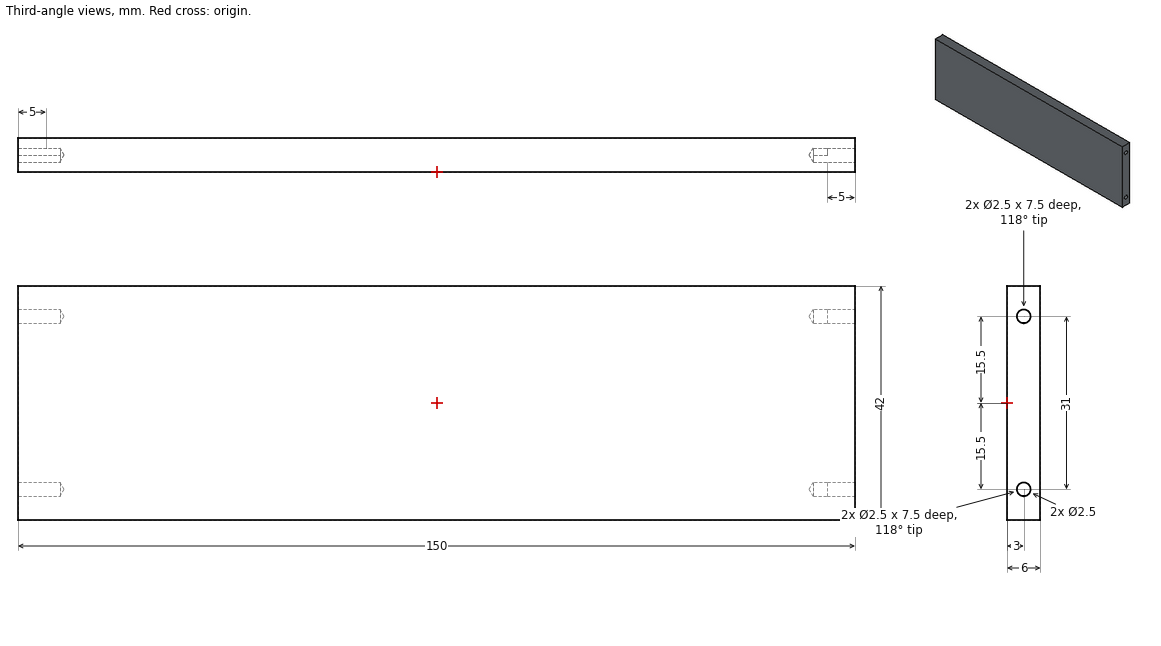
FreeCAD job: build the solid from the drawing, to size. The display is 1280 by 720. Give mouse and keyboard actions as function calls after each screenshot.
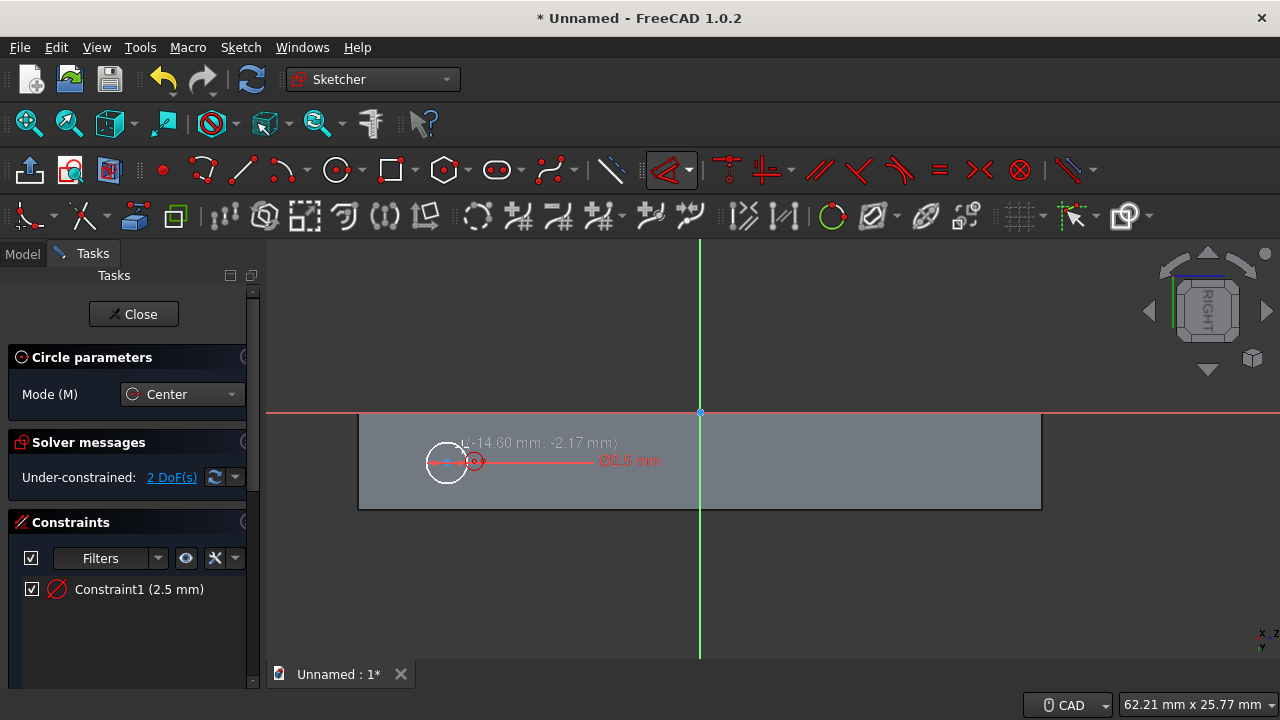
click(953, 462)
move(967, 447)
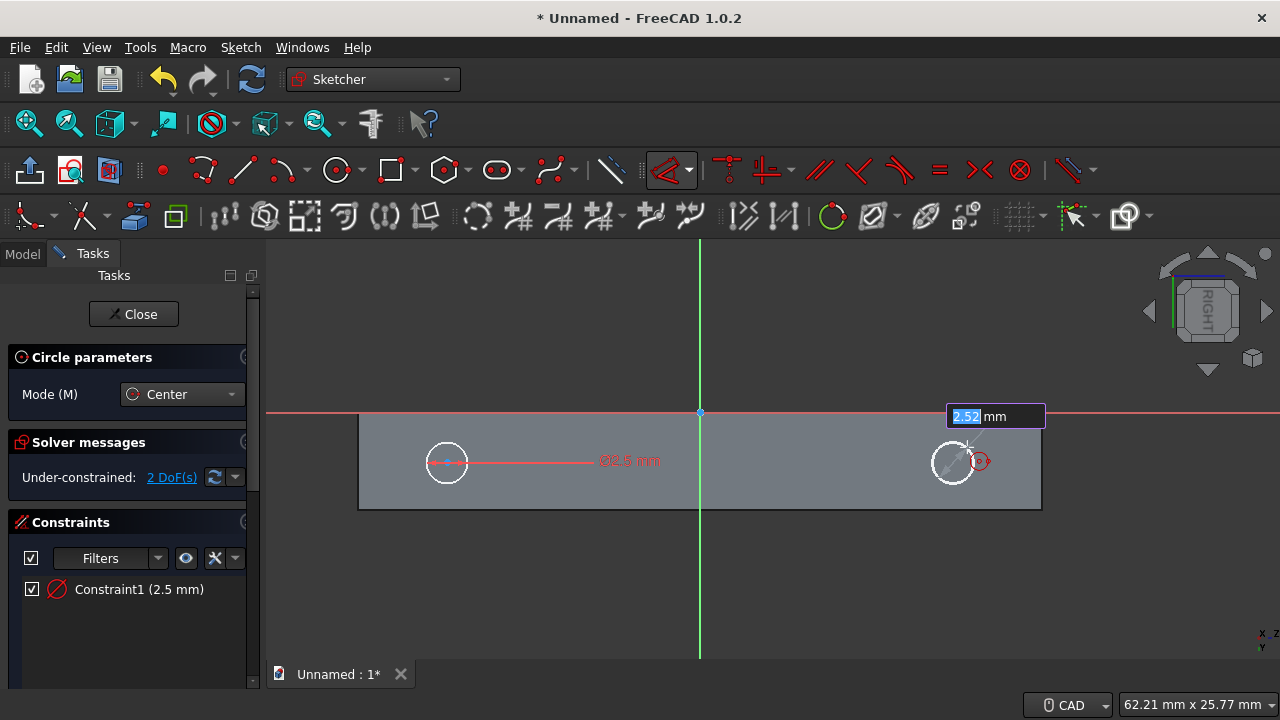
text(2.5)
key(Return)
key(Escape)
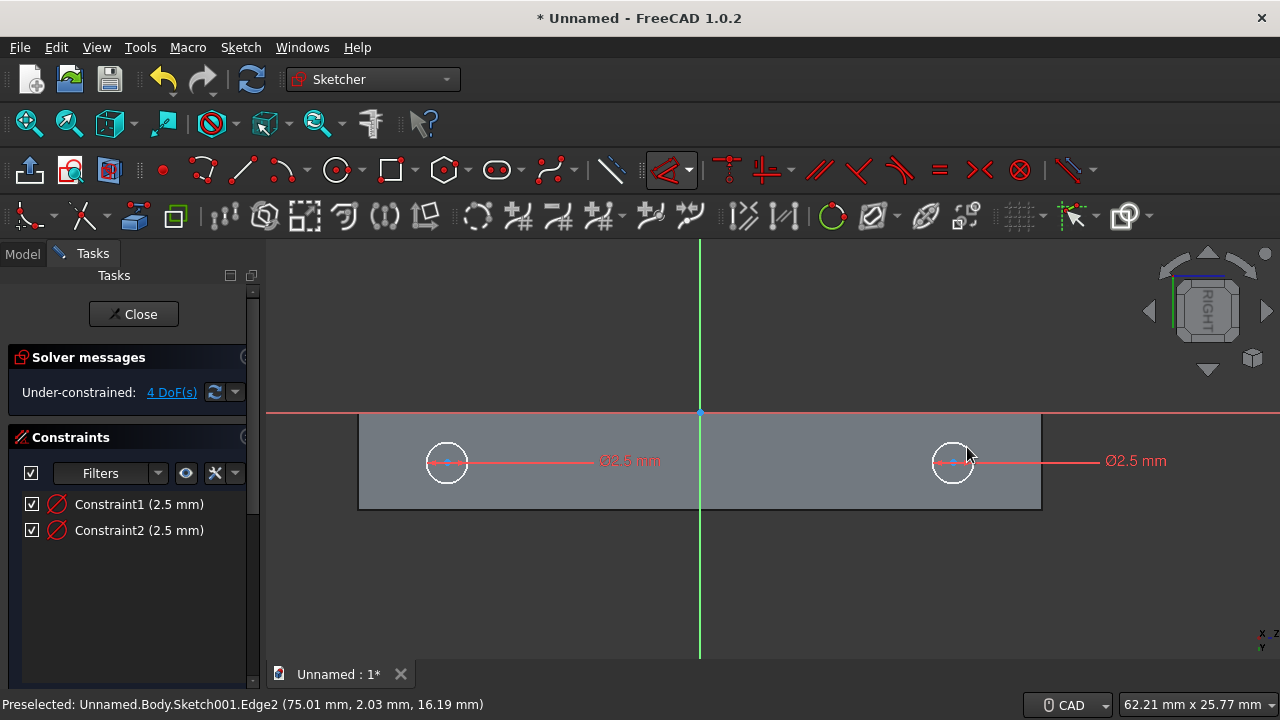
click(447, 463)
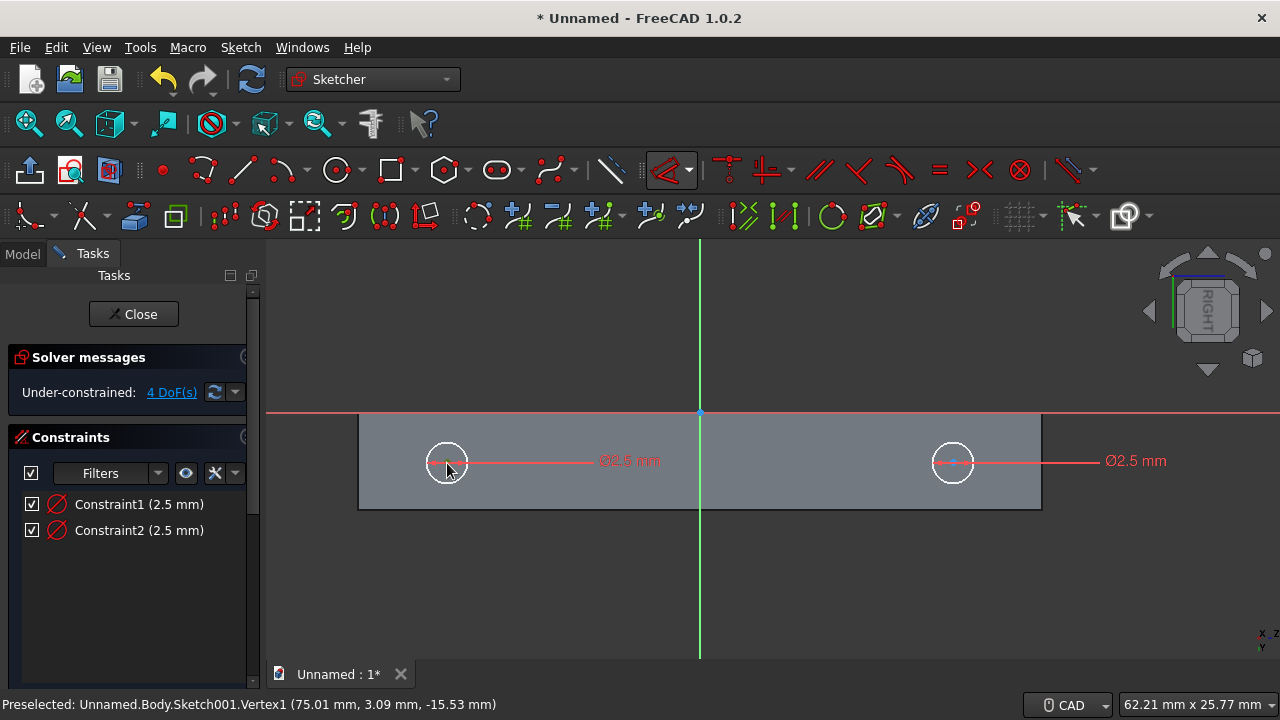
click(953, 463)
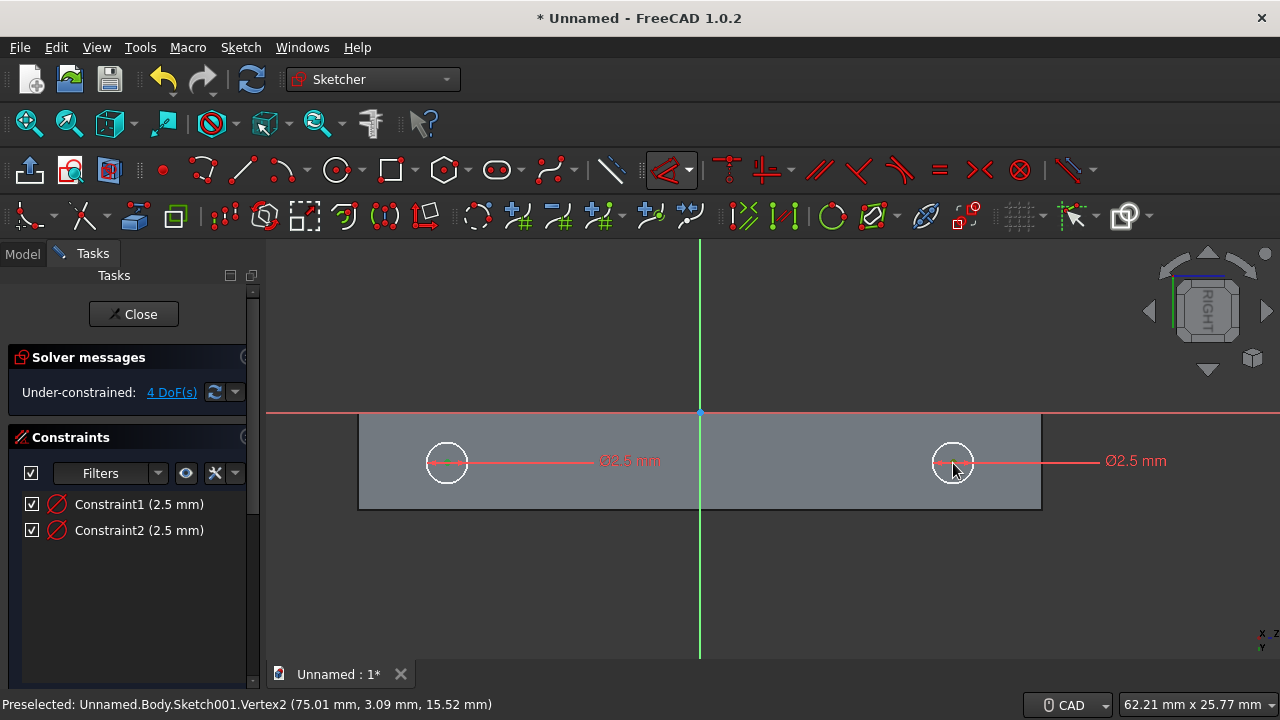
key(h)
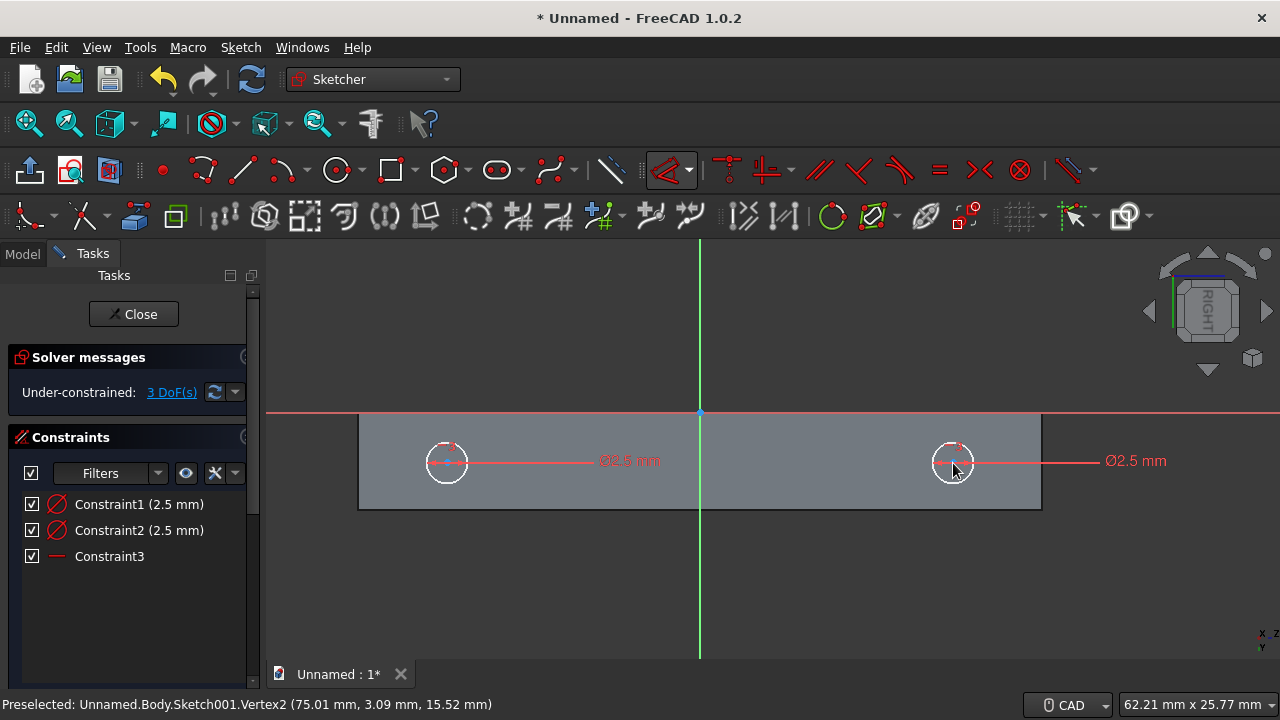
click(666, 170)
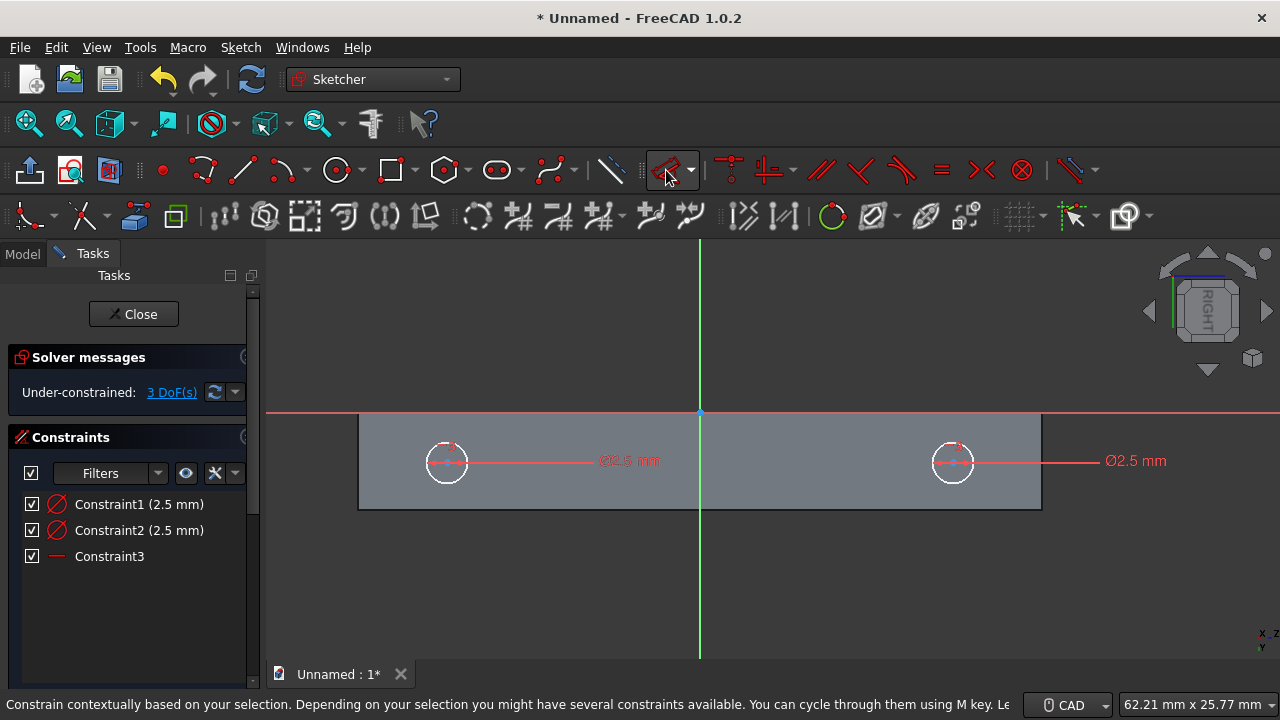
click(447, 463)
click(413, 438)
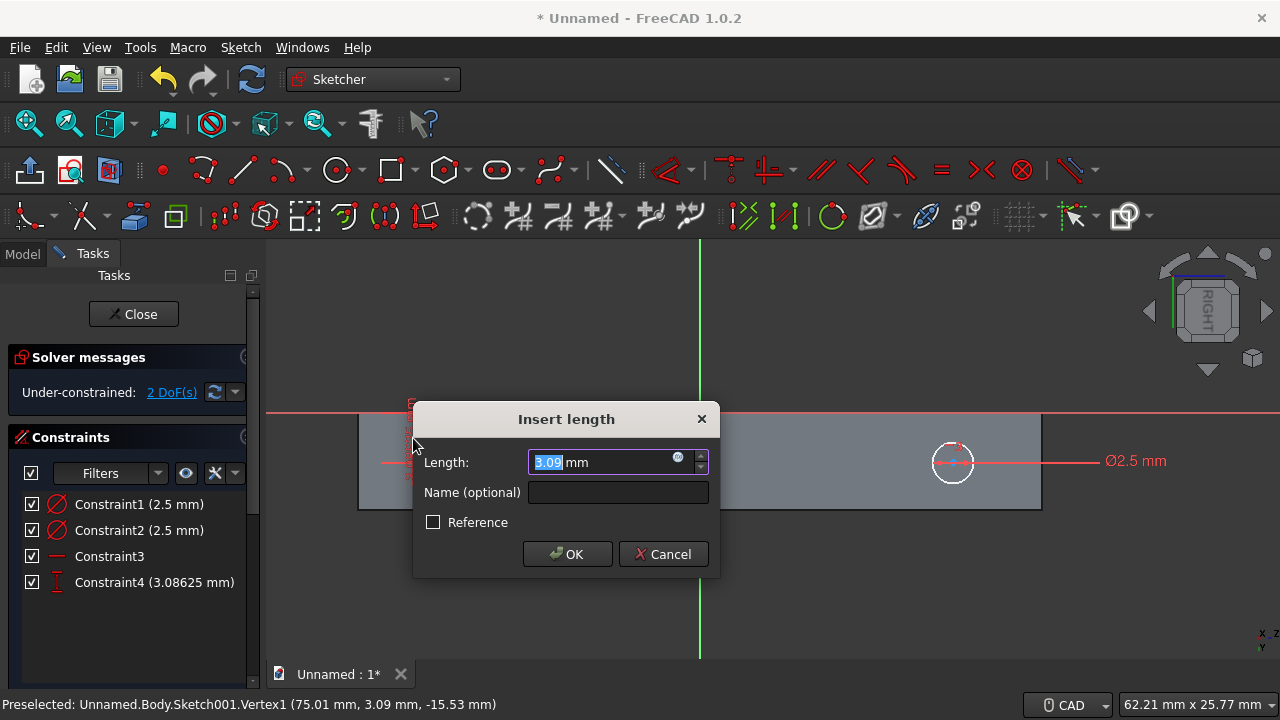
text(3)
key(Return)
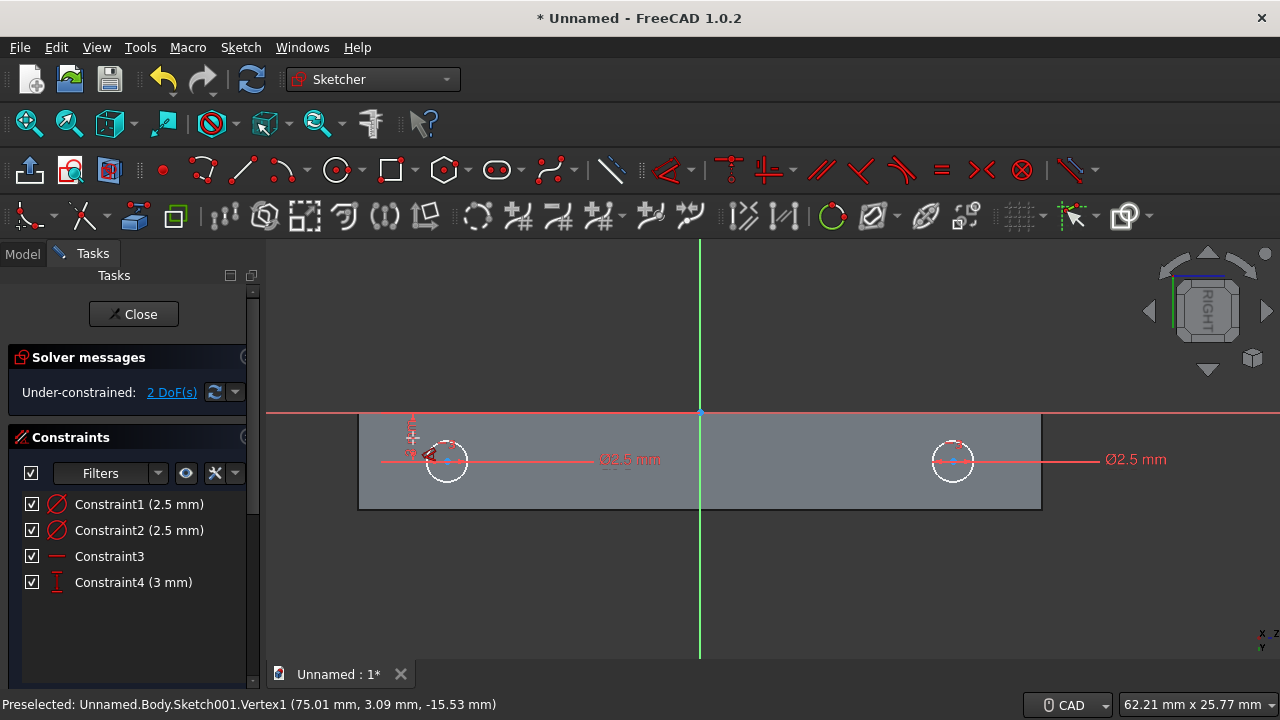
click(447, 462)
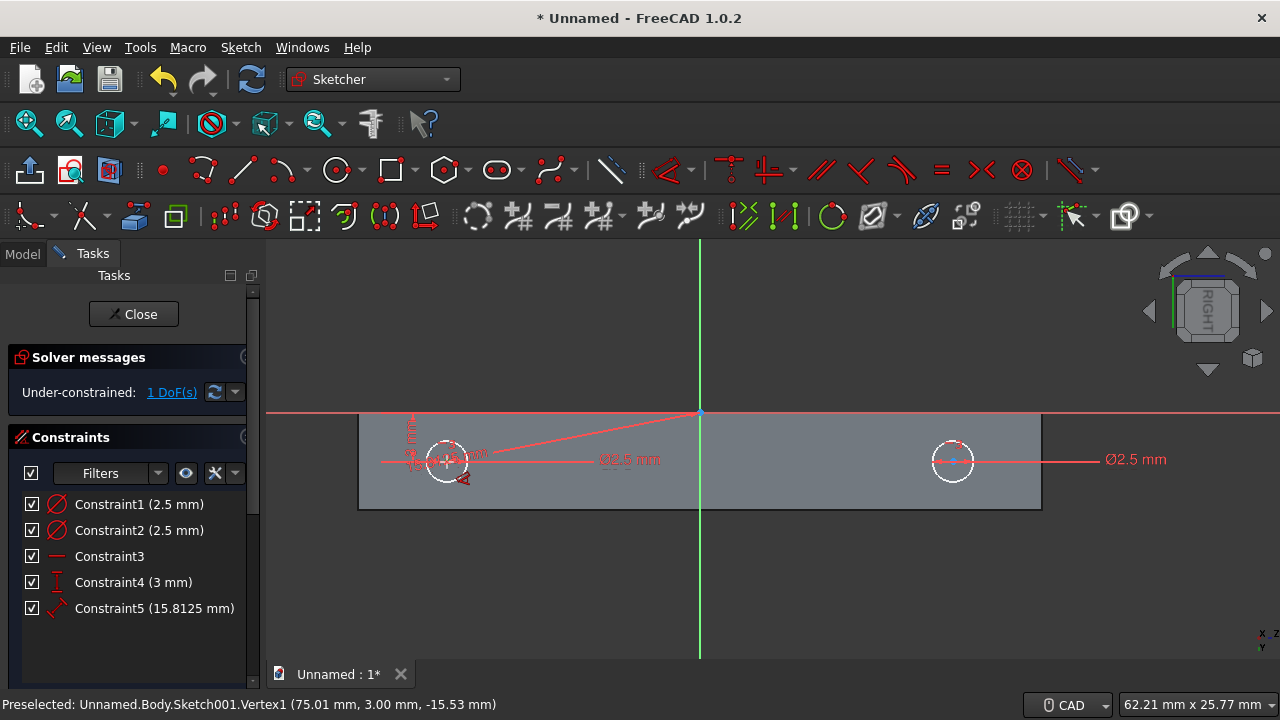
click(953, 462)
click(584, 496)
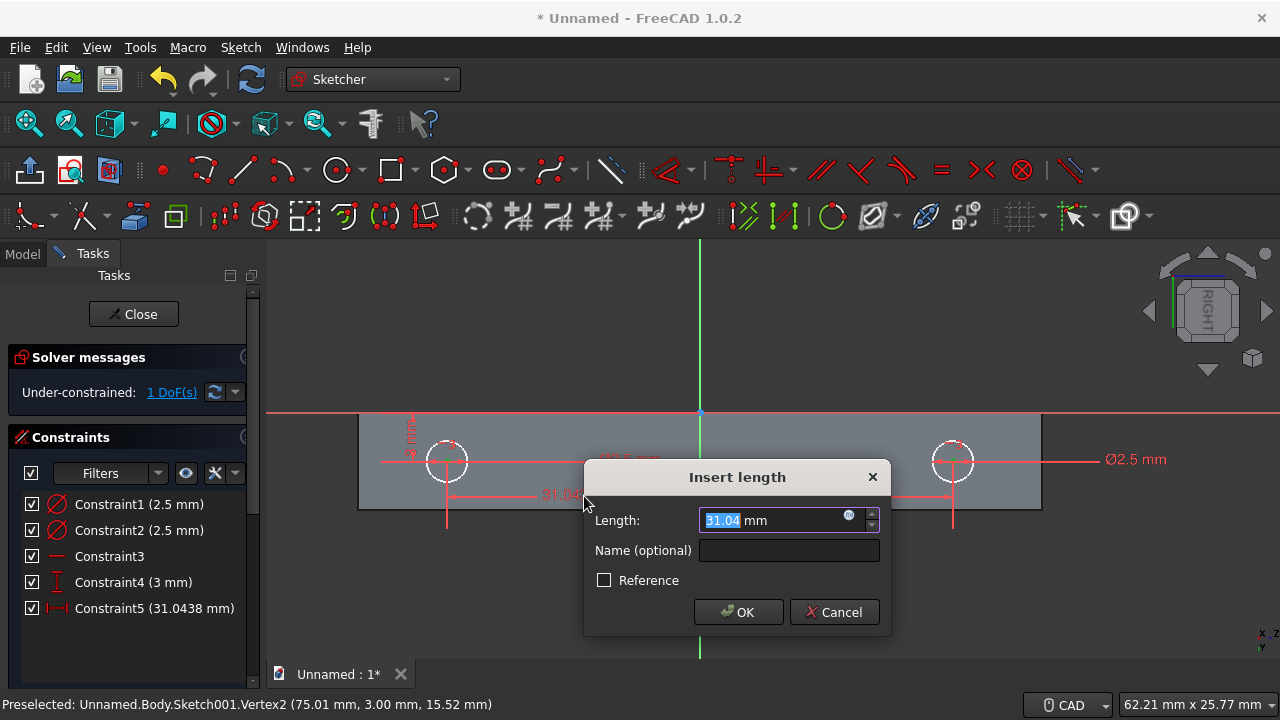
text(31)
key(Return)